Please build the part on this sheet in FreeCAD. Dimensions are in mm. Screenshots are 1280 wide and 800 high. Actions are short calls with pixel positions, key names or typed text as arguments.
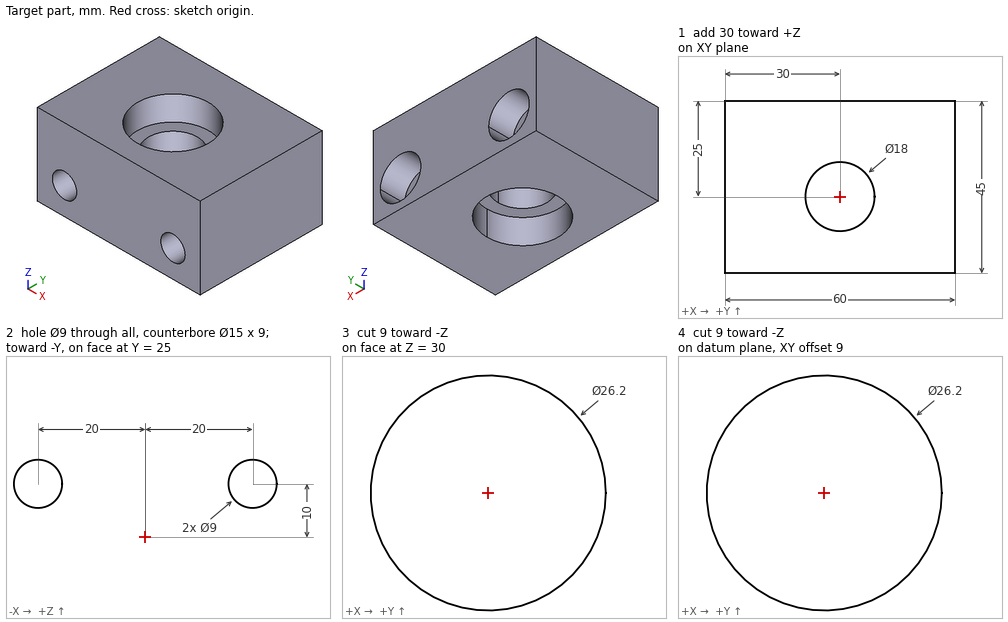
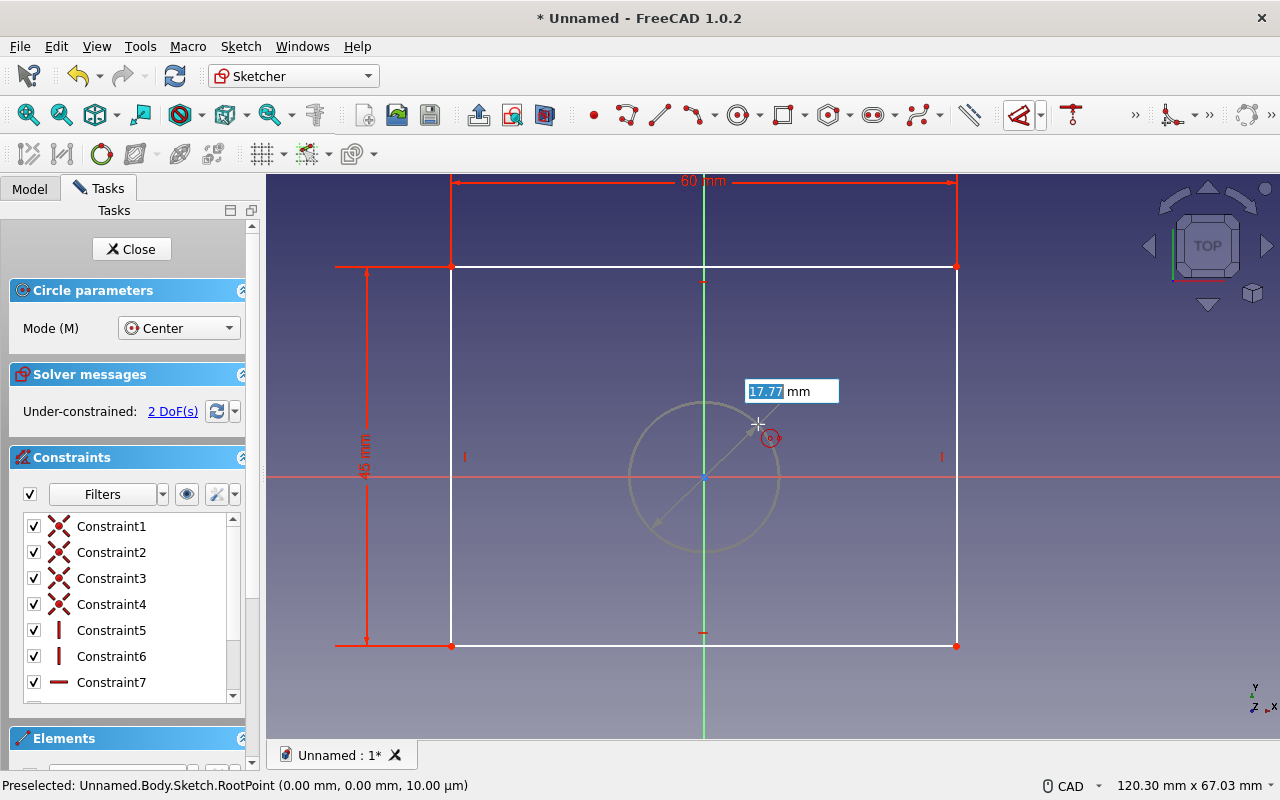
text(18)
key(Return)
key(Escape)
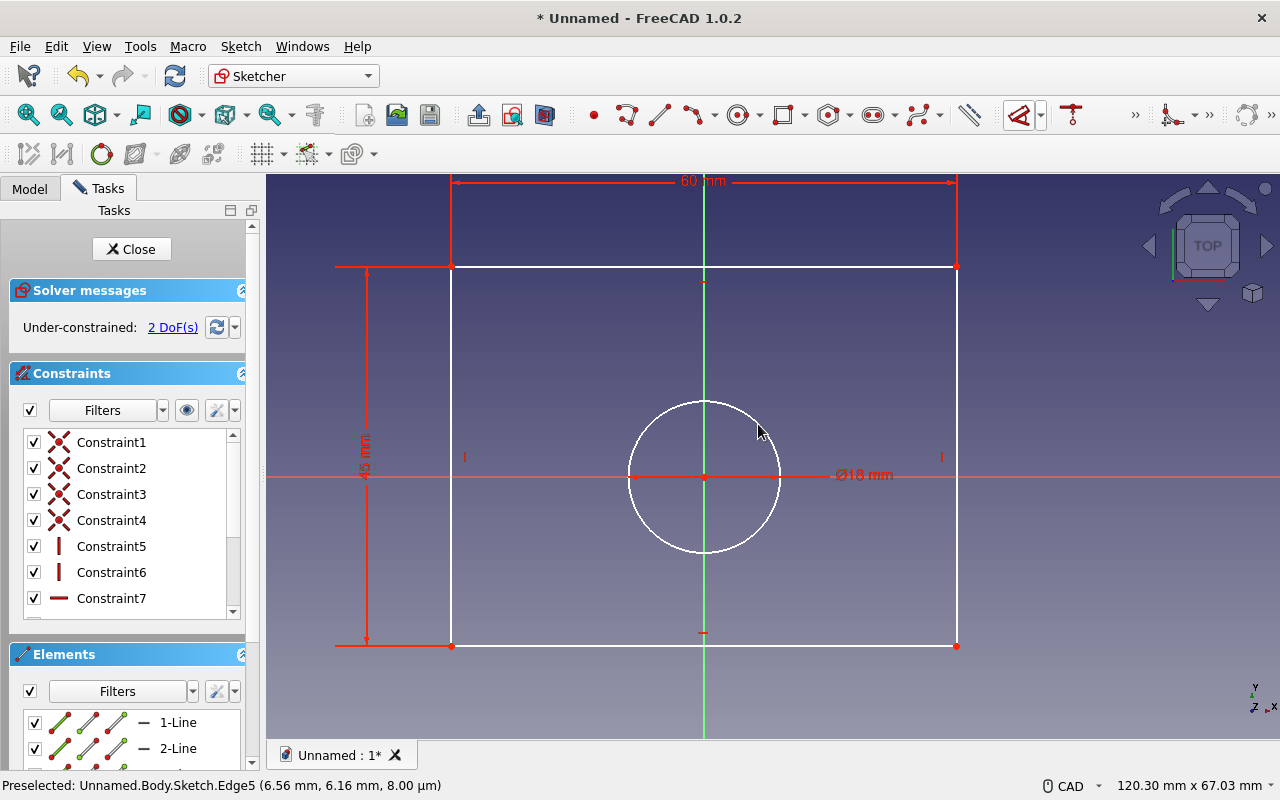
click(451, 267)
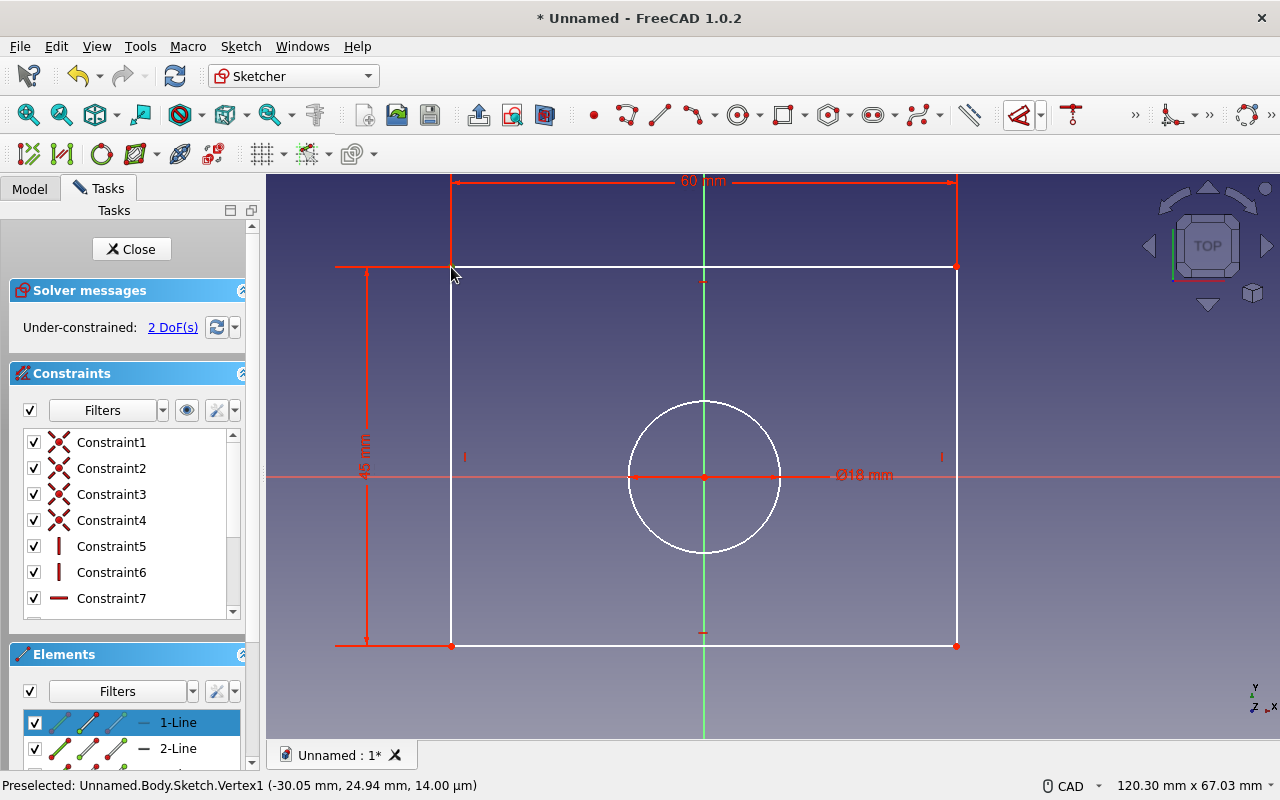
click(1040, 116)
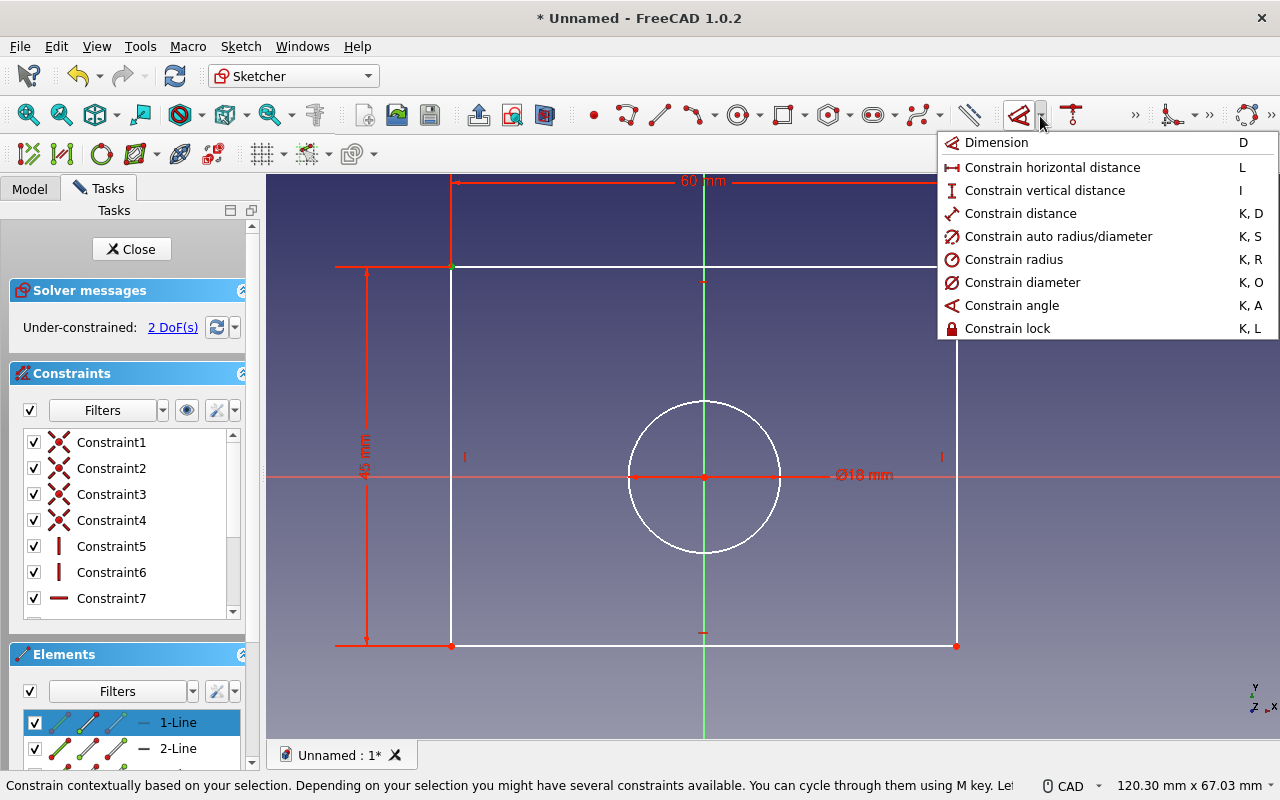
click(1108, 168)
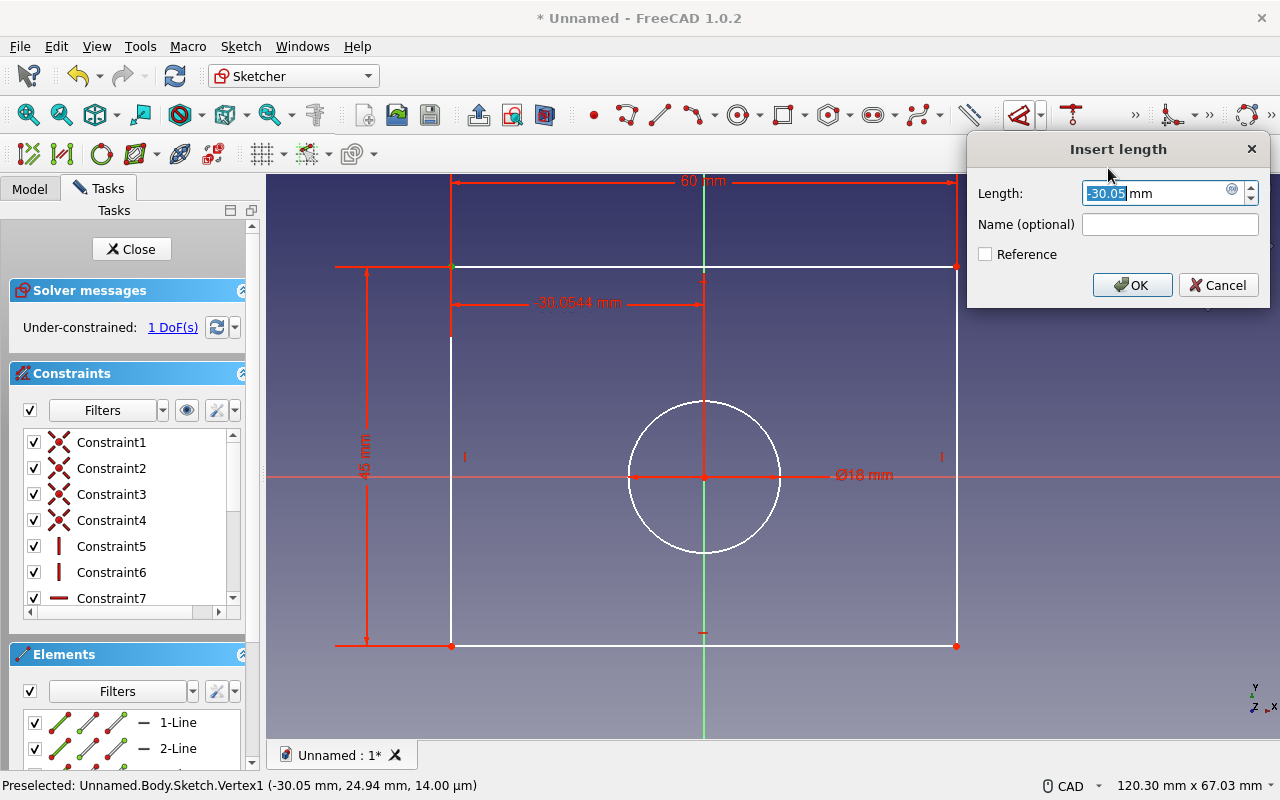
text(-30)
key(Return)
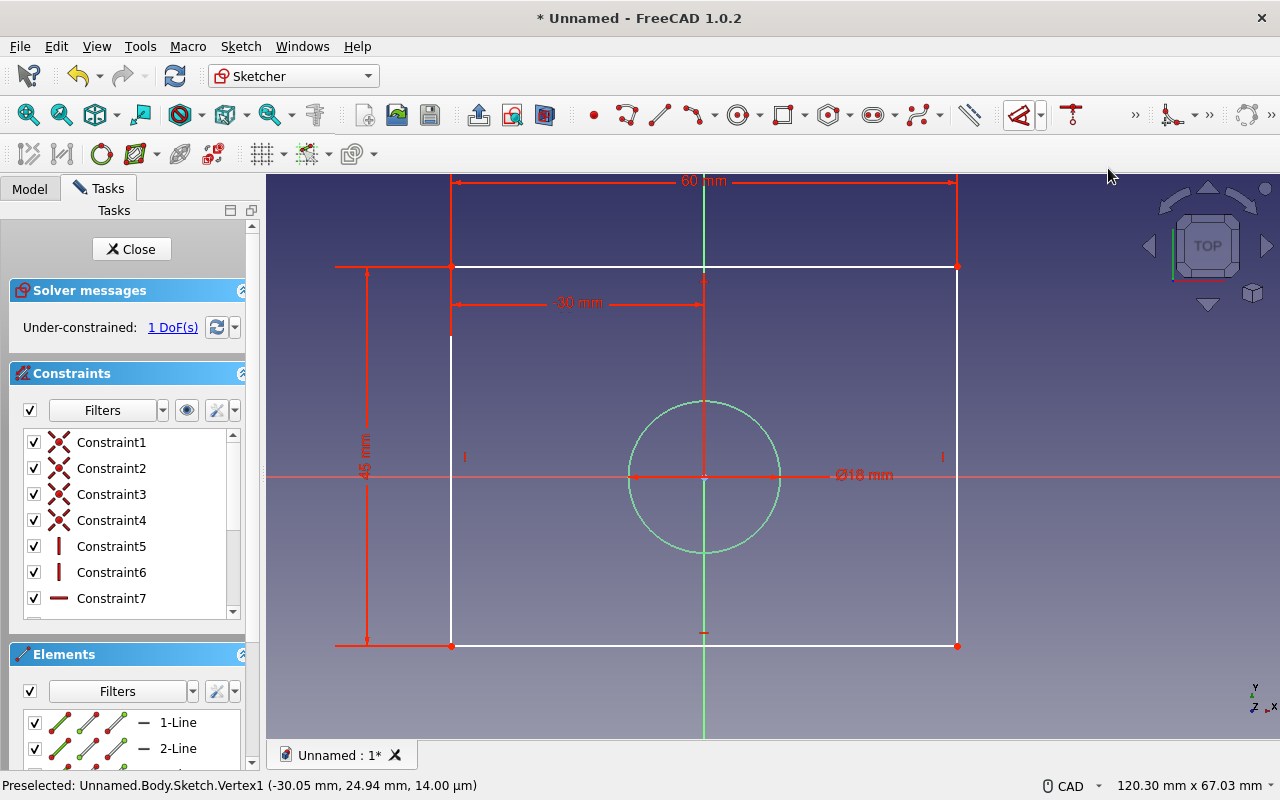
click(451, 267)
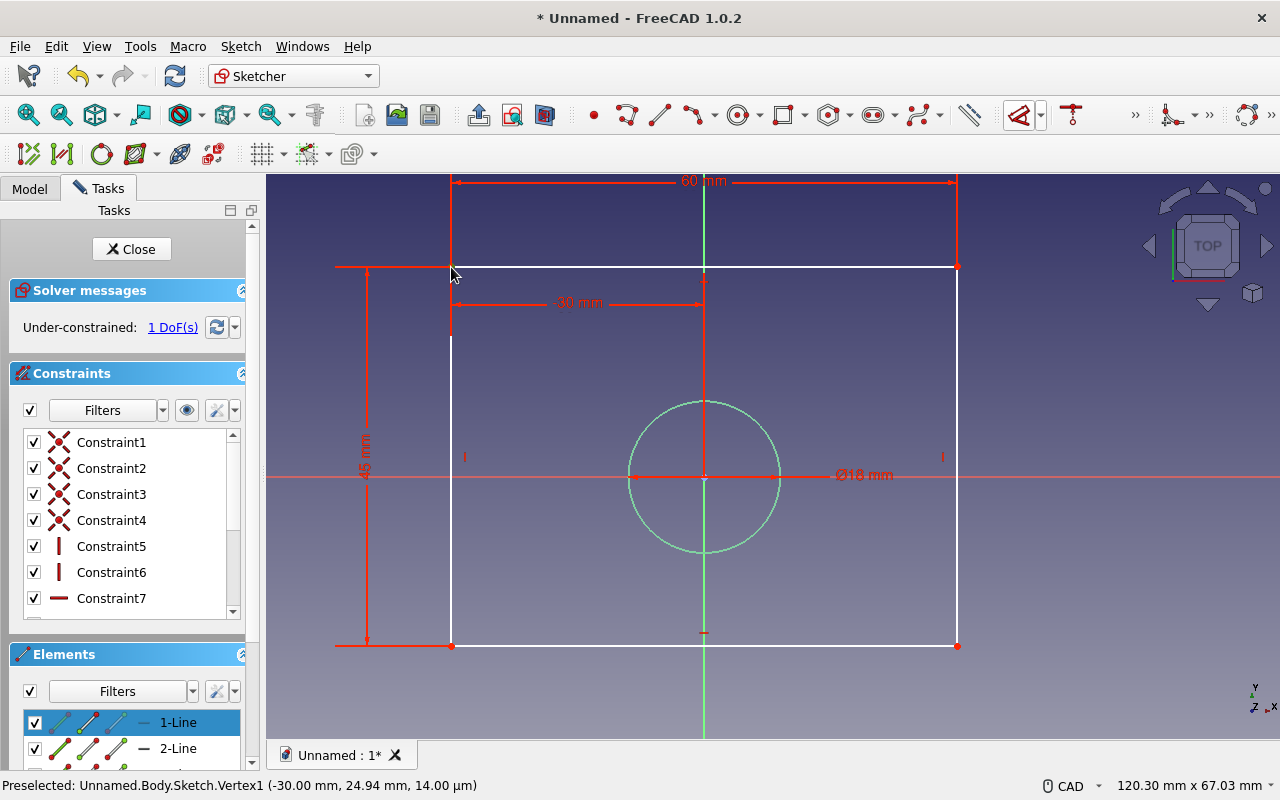
key(i)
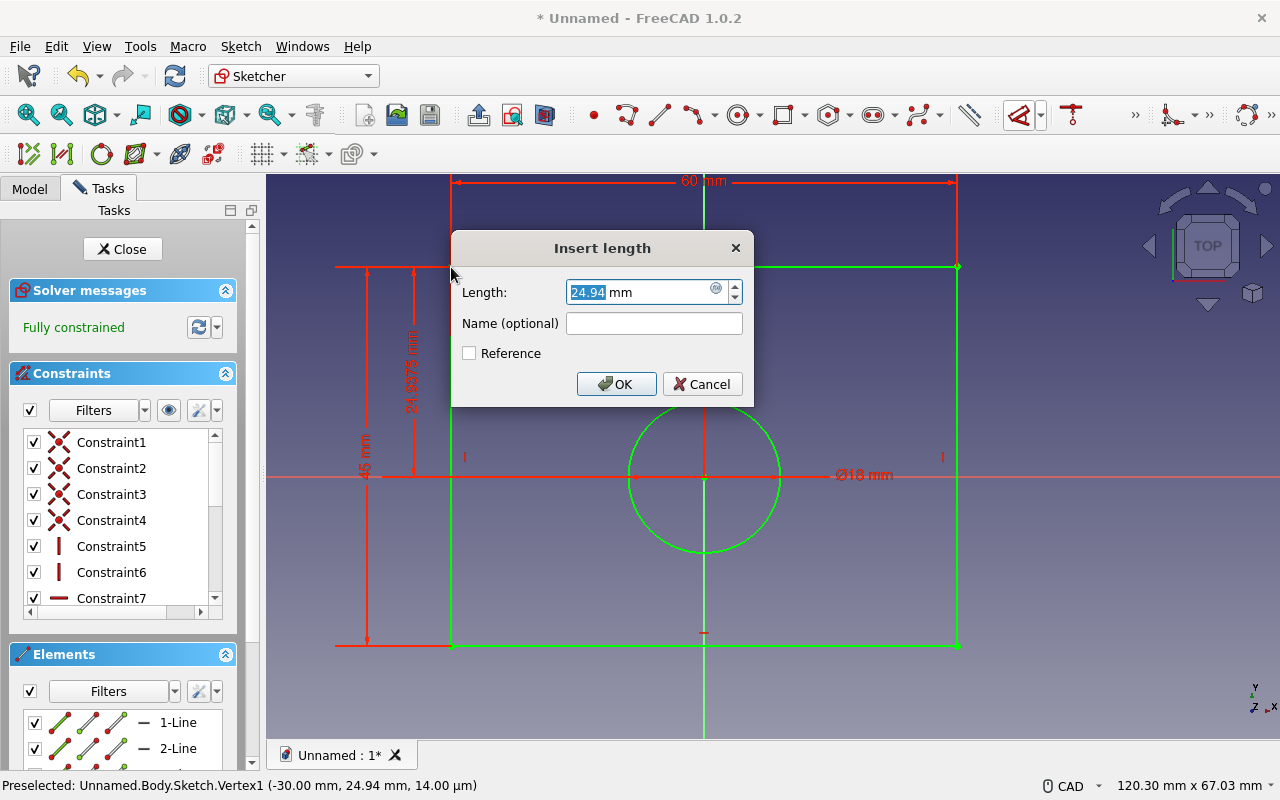
text(25)
key(Return)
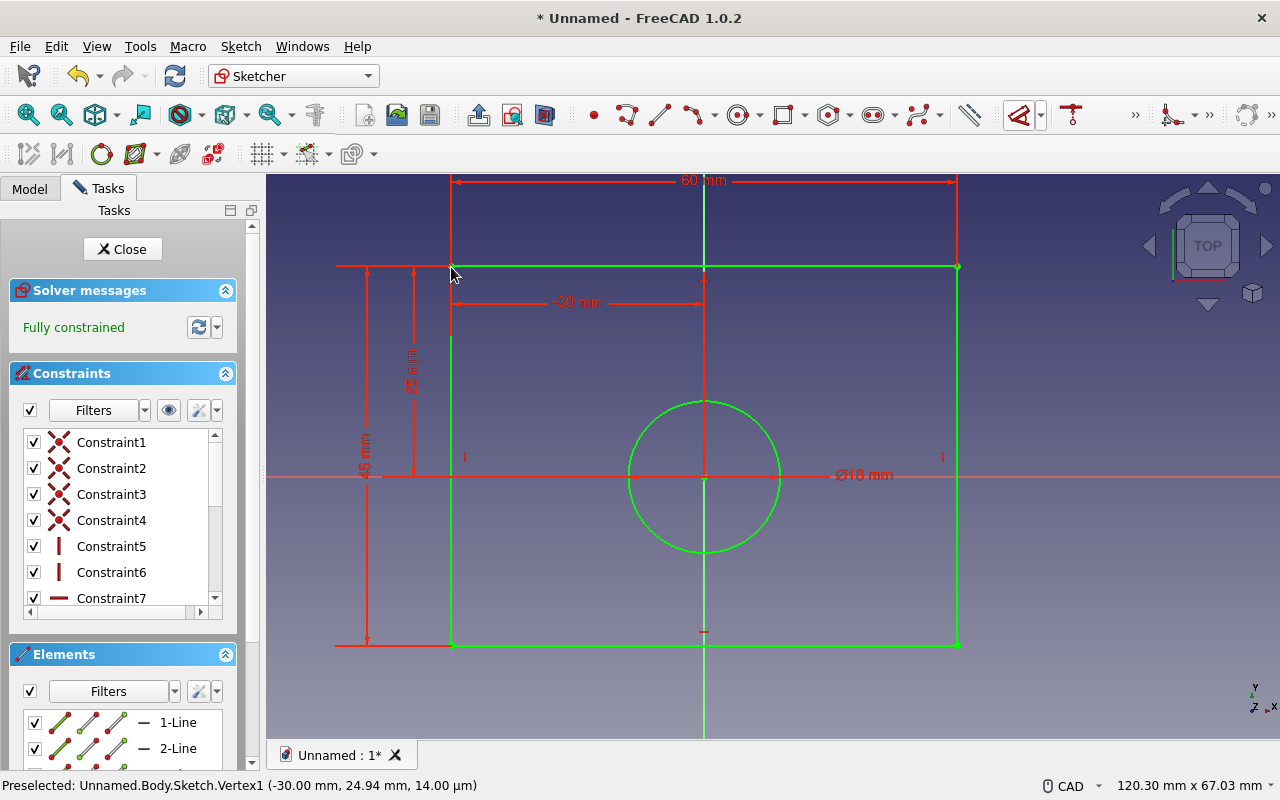
click(123, 249)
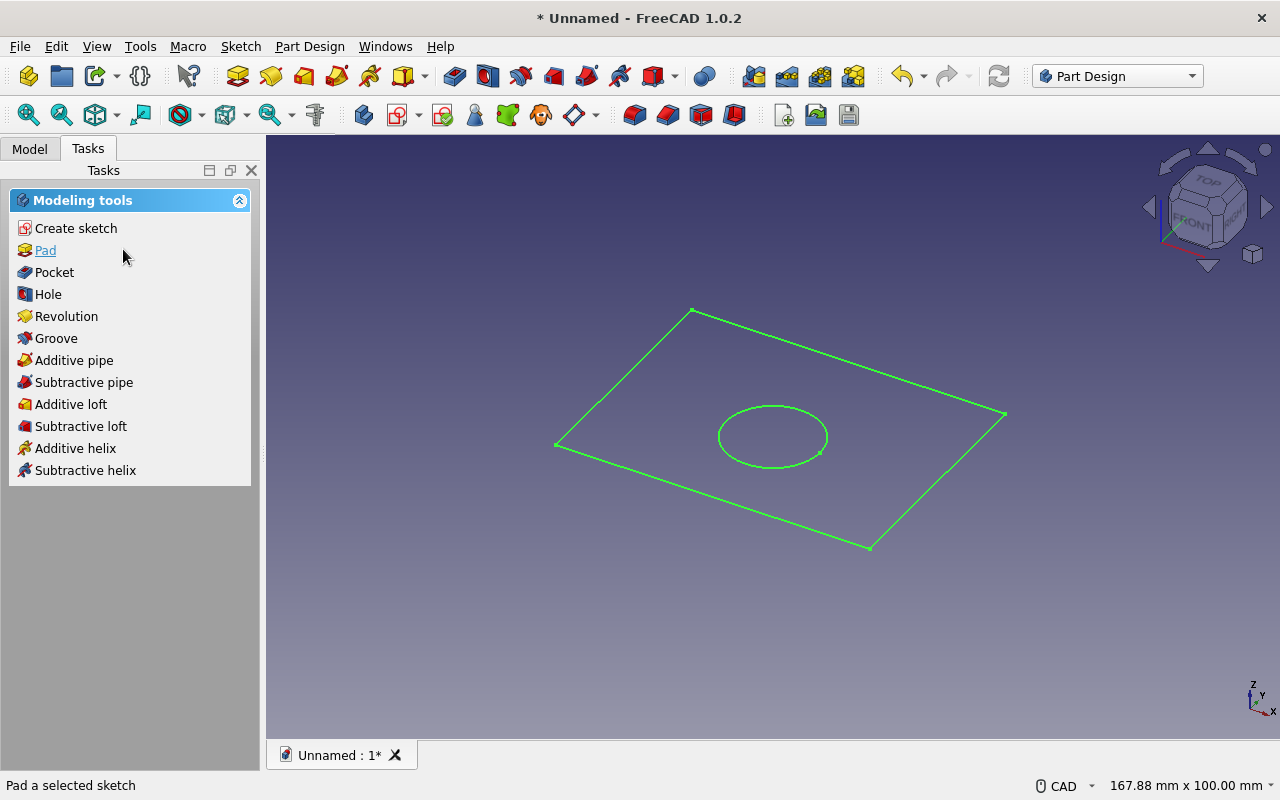
click(238, 76)